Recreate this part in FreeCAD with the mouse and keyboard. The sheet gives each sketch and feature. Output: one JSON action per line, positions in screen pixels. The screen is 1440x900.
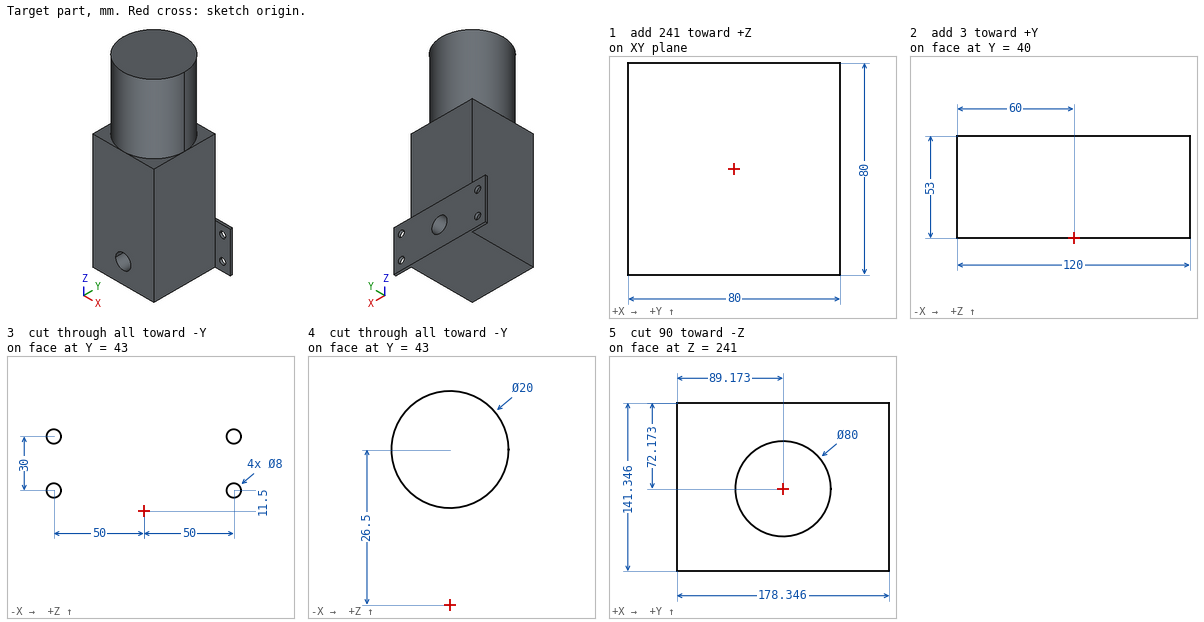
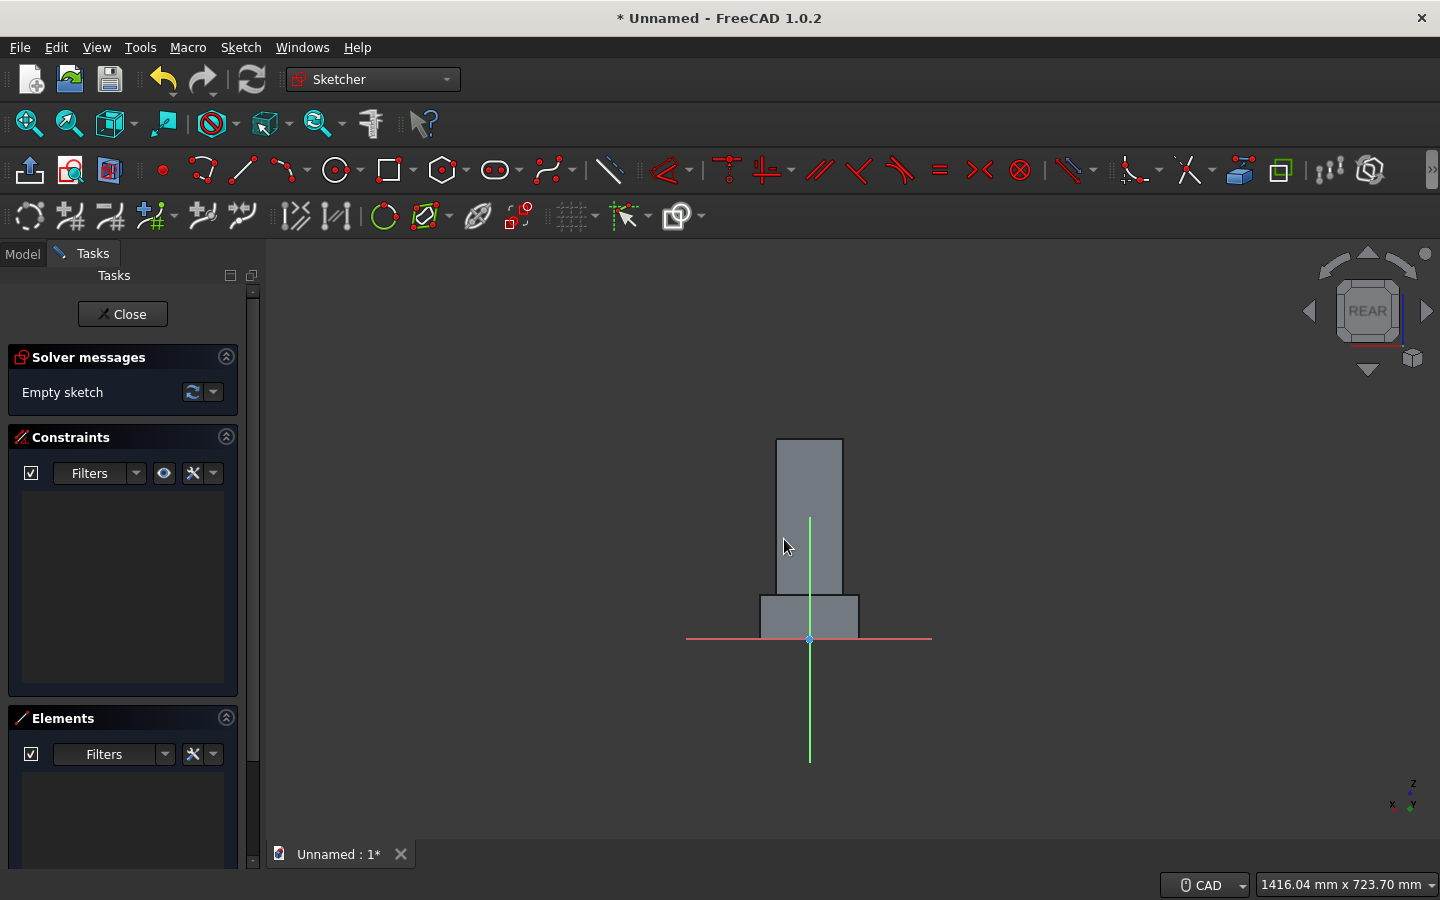
{"action": "scroll", "coordinate": [814, 633], "scroll_direction": "up", "scroll_amount": 10}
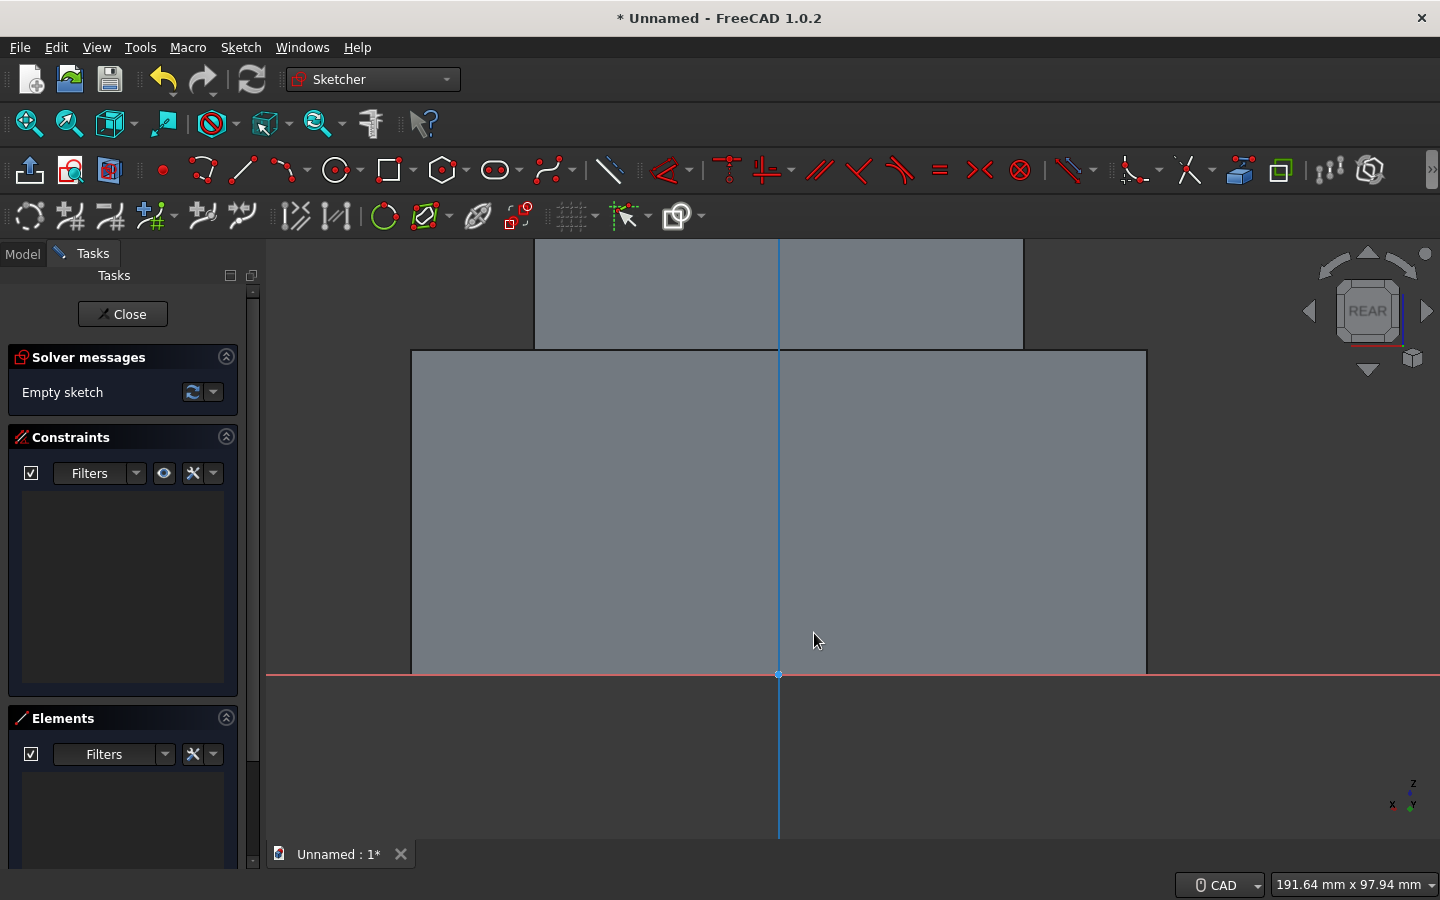
{"action": "left_click", "coordinate": [336, 170]}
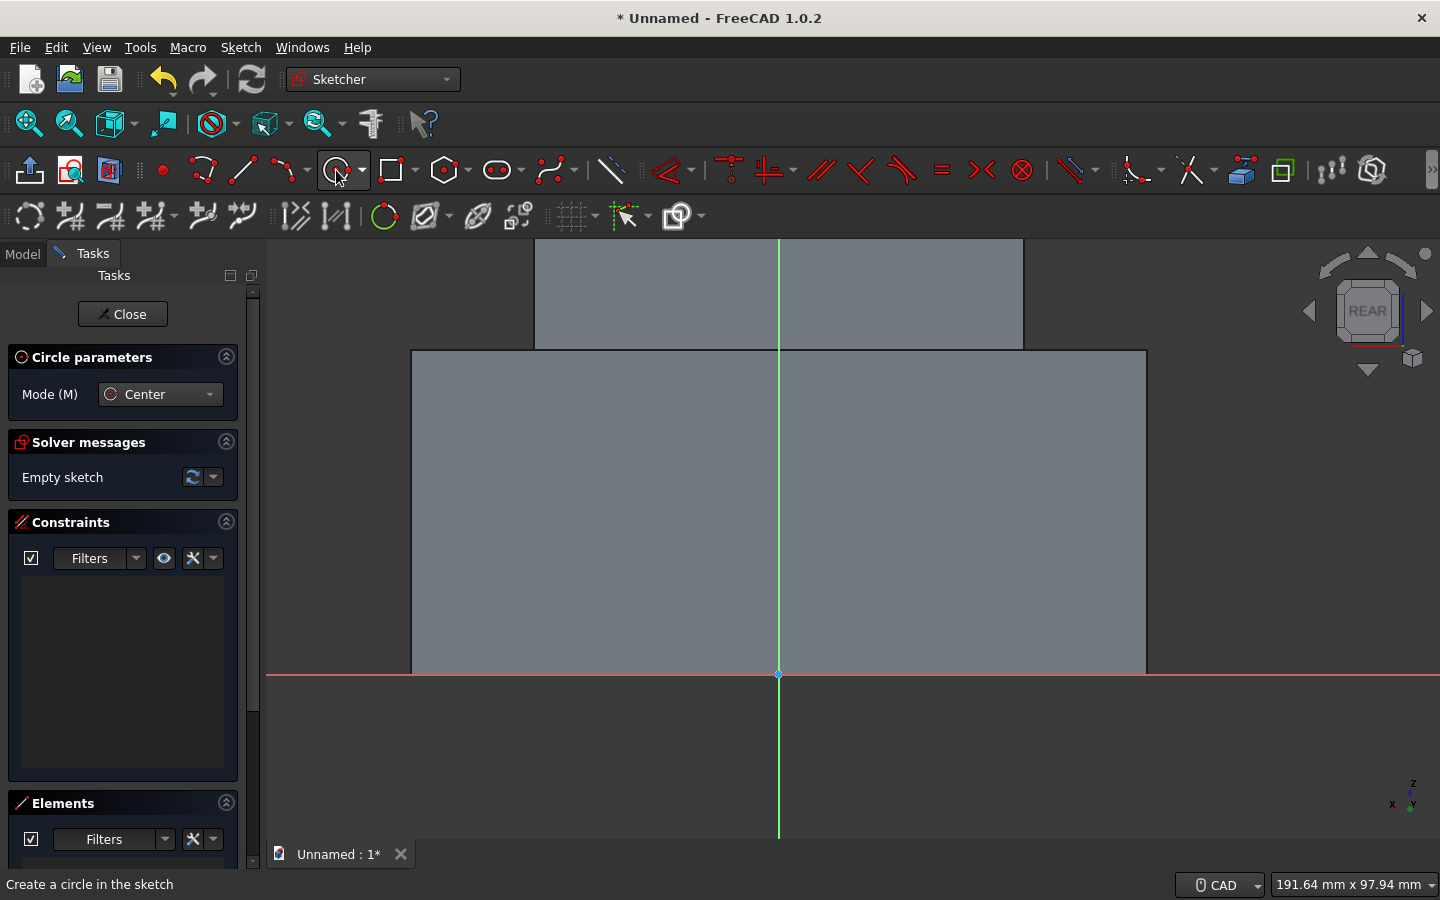
{"action": "left_click", "coordinate": [1085, 604]}
{"action": "left_click", "coordinate": [1103, 587]}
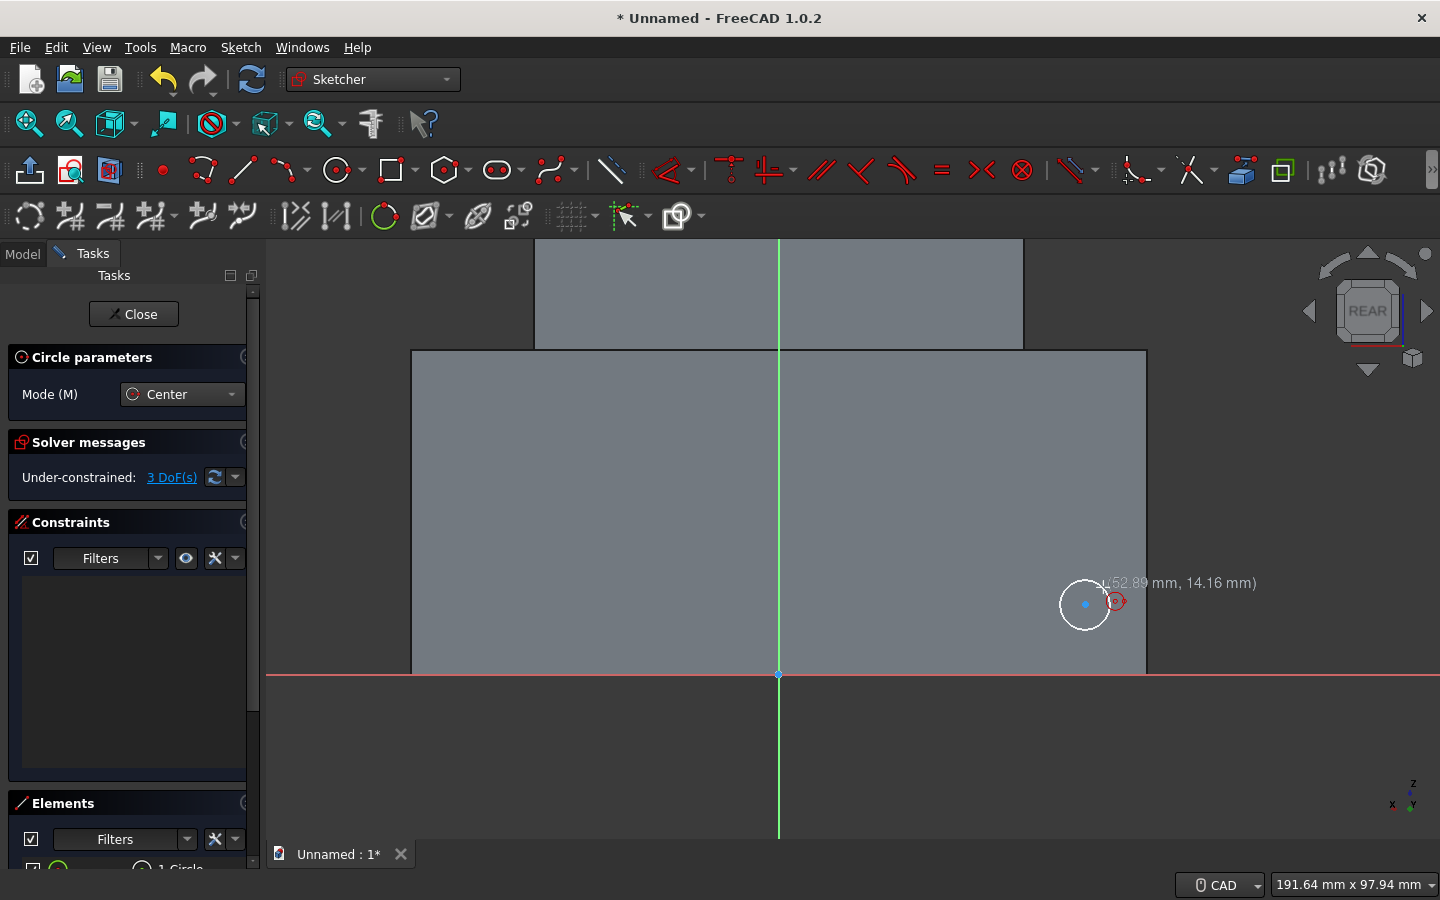
{"action": "left_click", "coordinate": [473, 604]}
{"action": "left_click", "coordinate": [490, 587]}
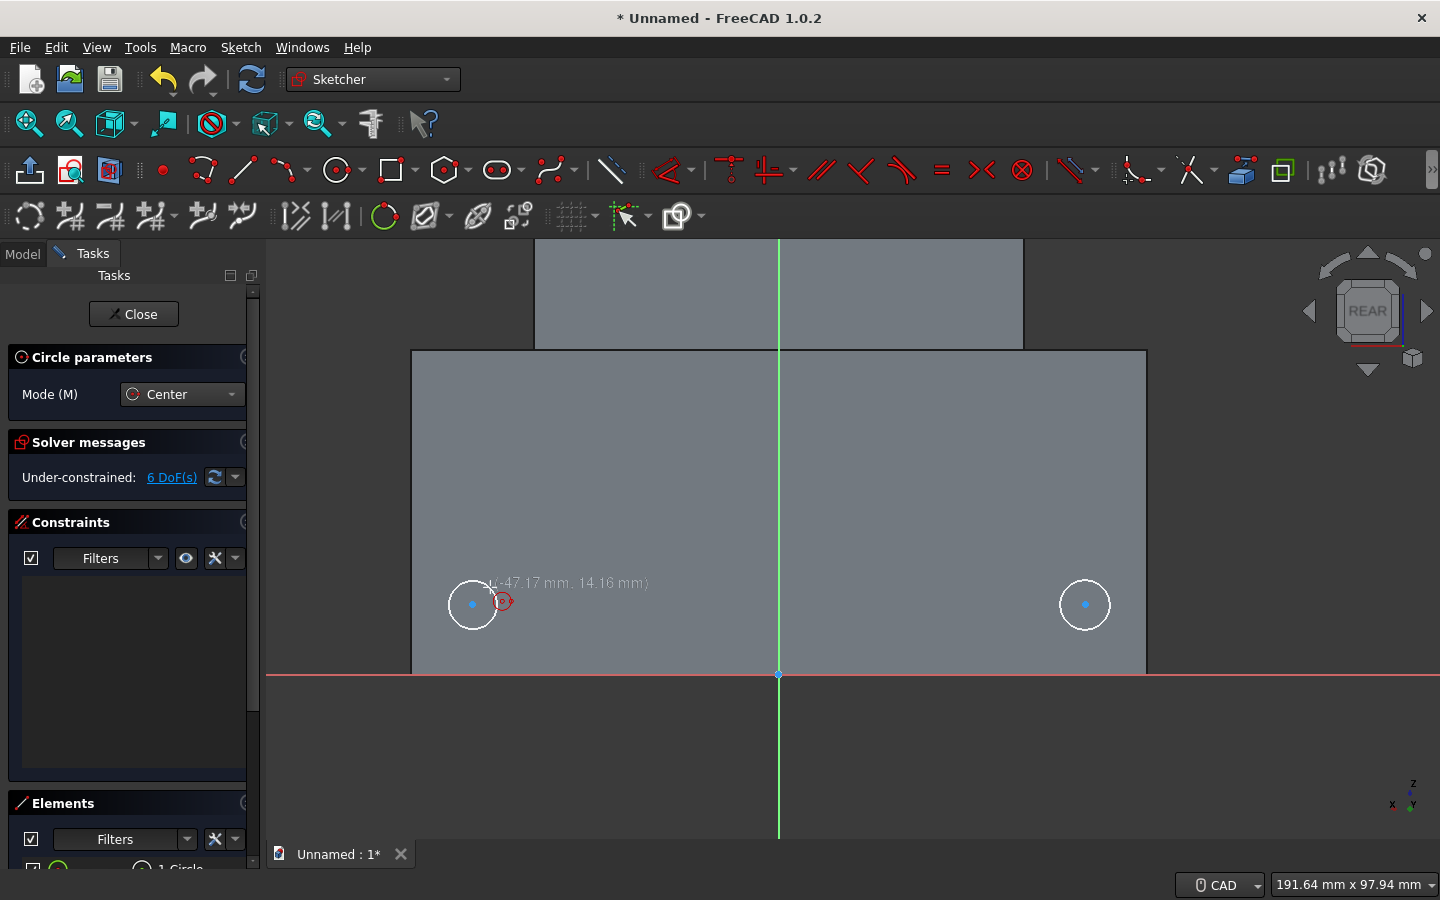
{"action": "left_click", "coordinate": [473, 421]}
{"action": "left_click", "coordinate": [490, 403]}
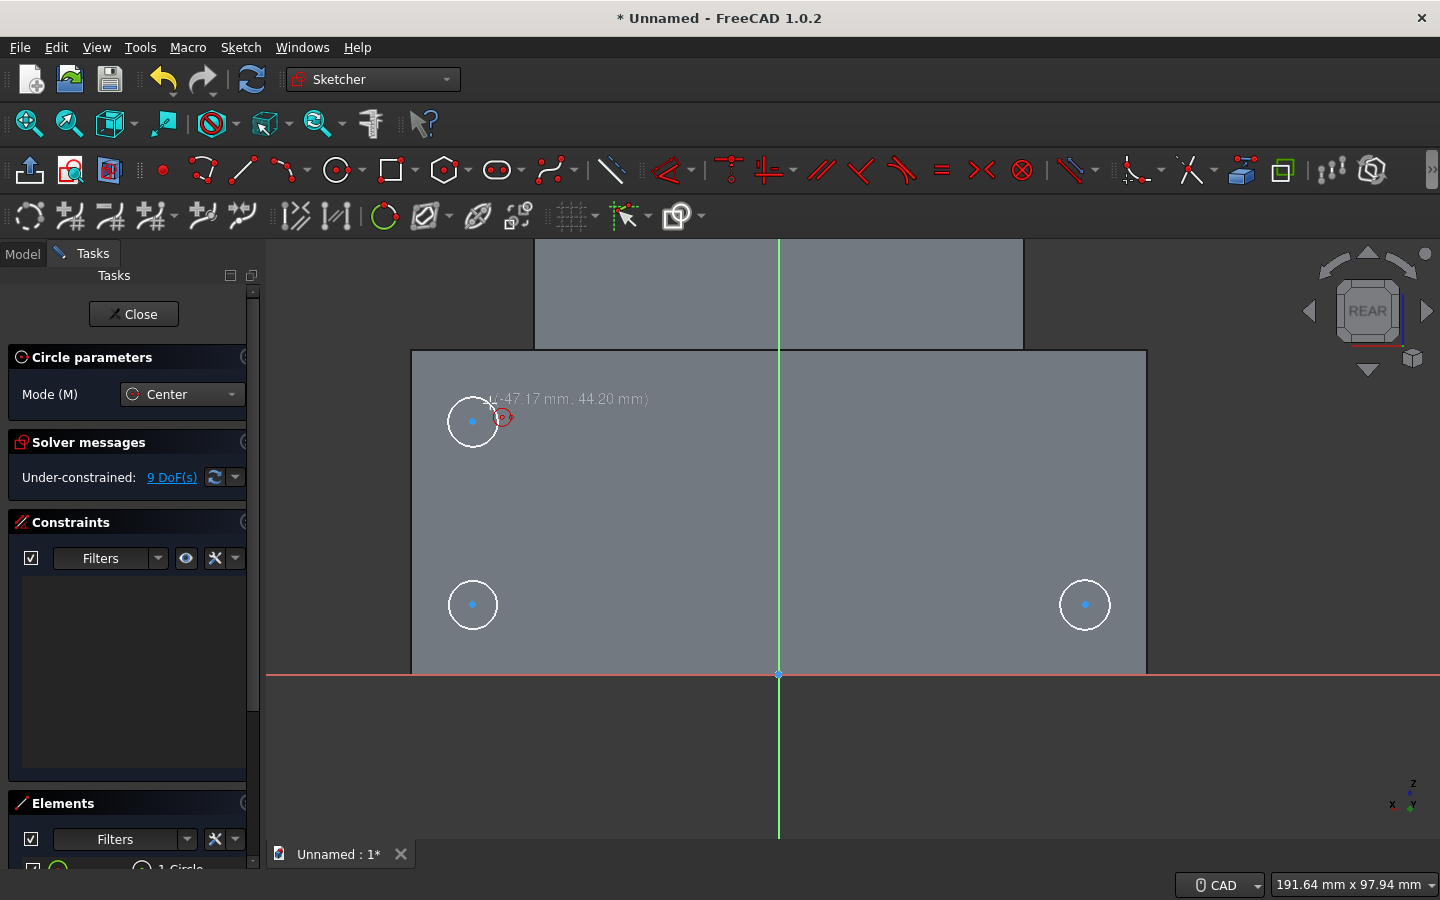
{"action": "left_click", "coordinate": [1085, 421]}
{"action": "left_click", "coordinate": [1103, 403]}
{"action": "key", "text": "Escape"}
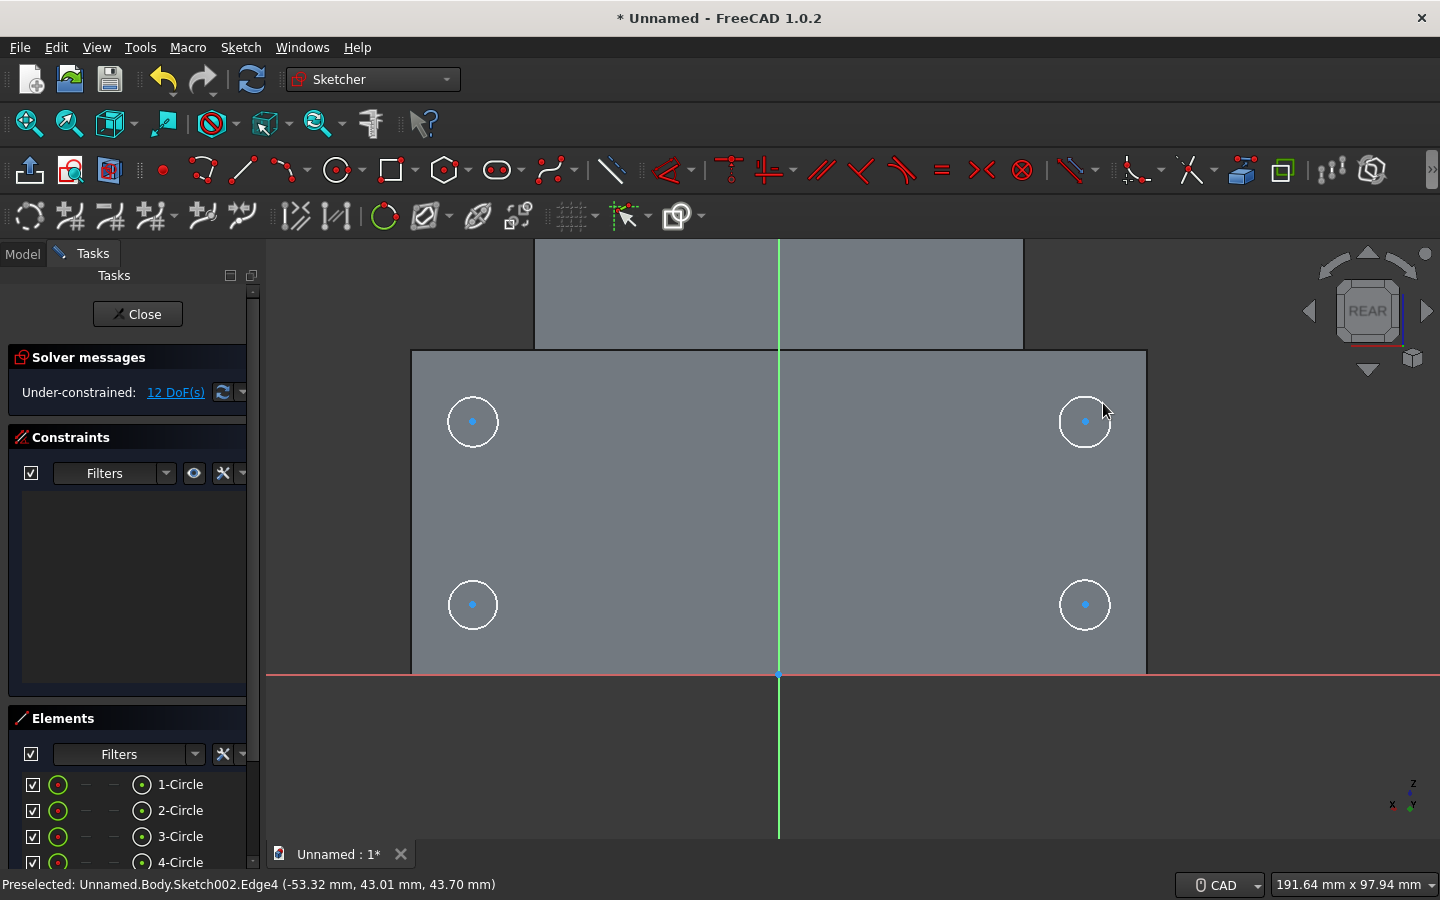
{"action": "left_click", "coordinate": [1102, 587]}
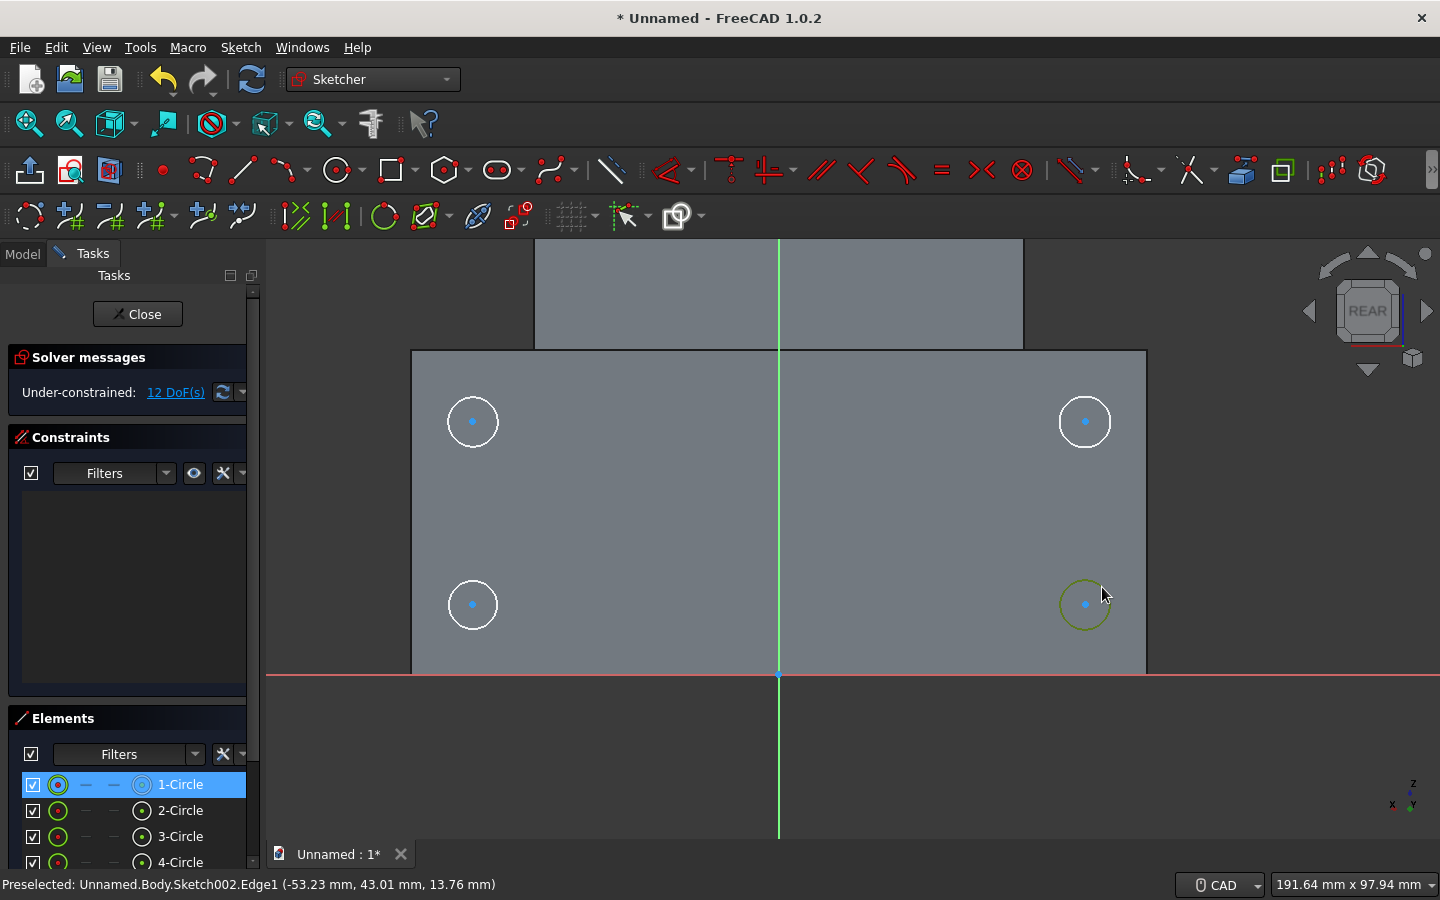
{"action": "left_click", "coordinate": [490, 588]}